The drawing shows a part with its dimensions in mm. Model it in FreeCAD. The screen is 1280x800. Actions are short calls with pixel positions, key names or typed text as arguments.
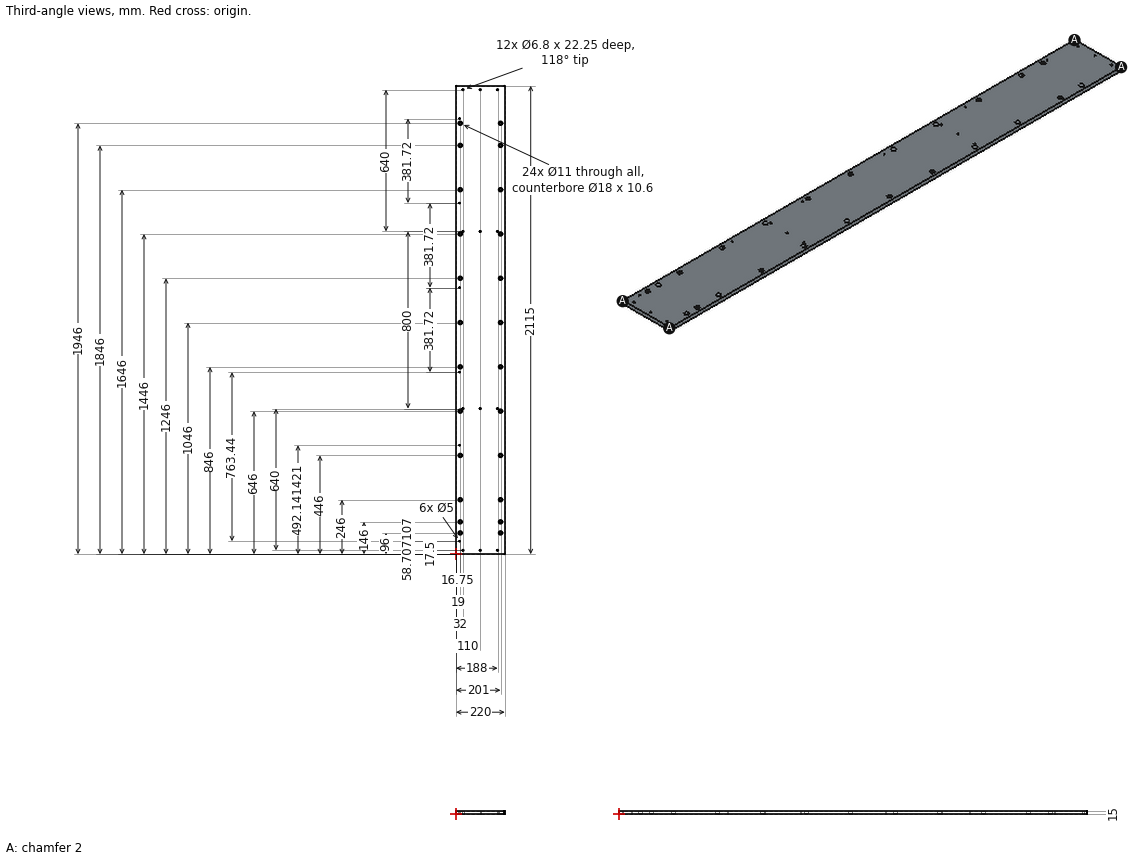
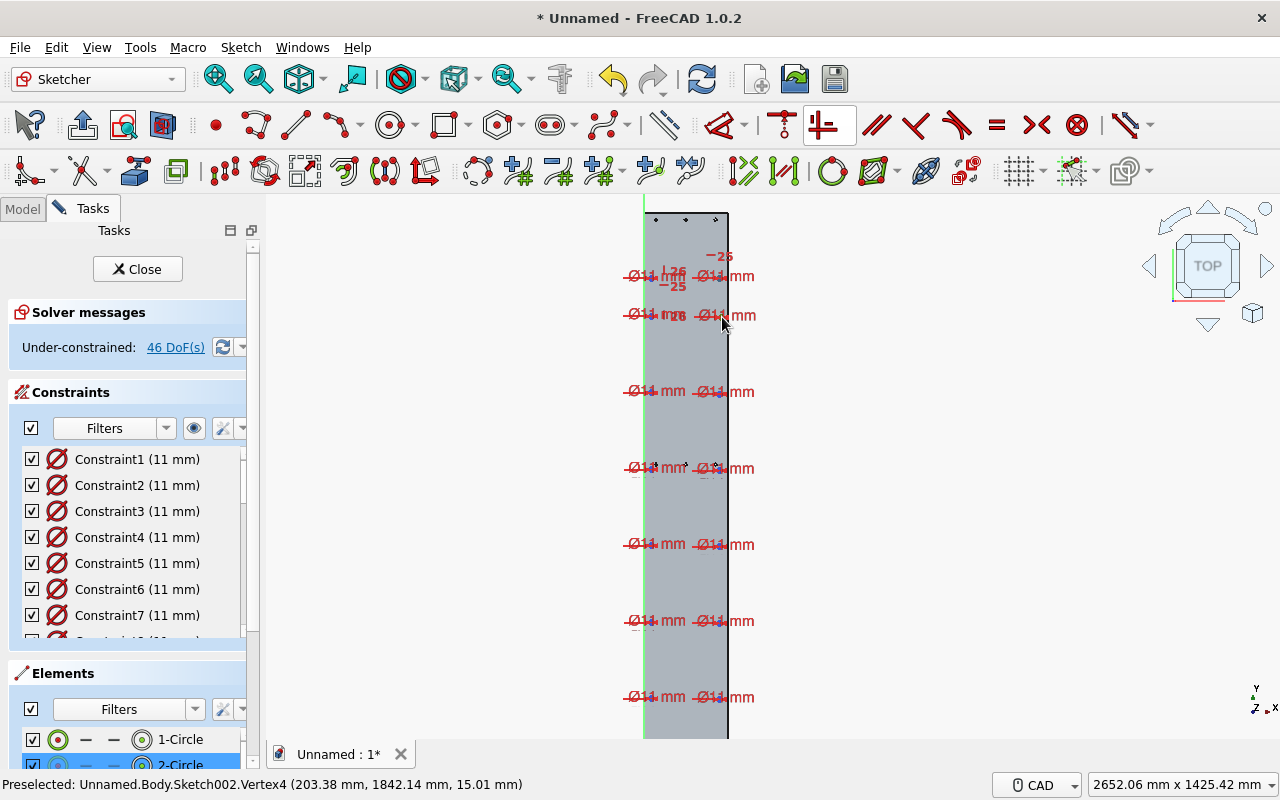
click(850, 126)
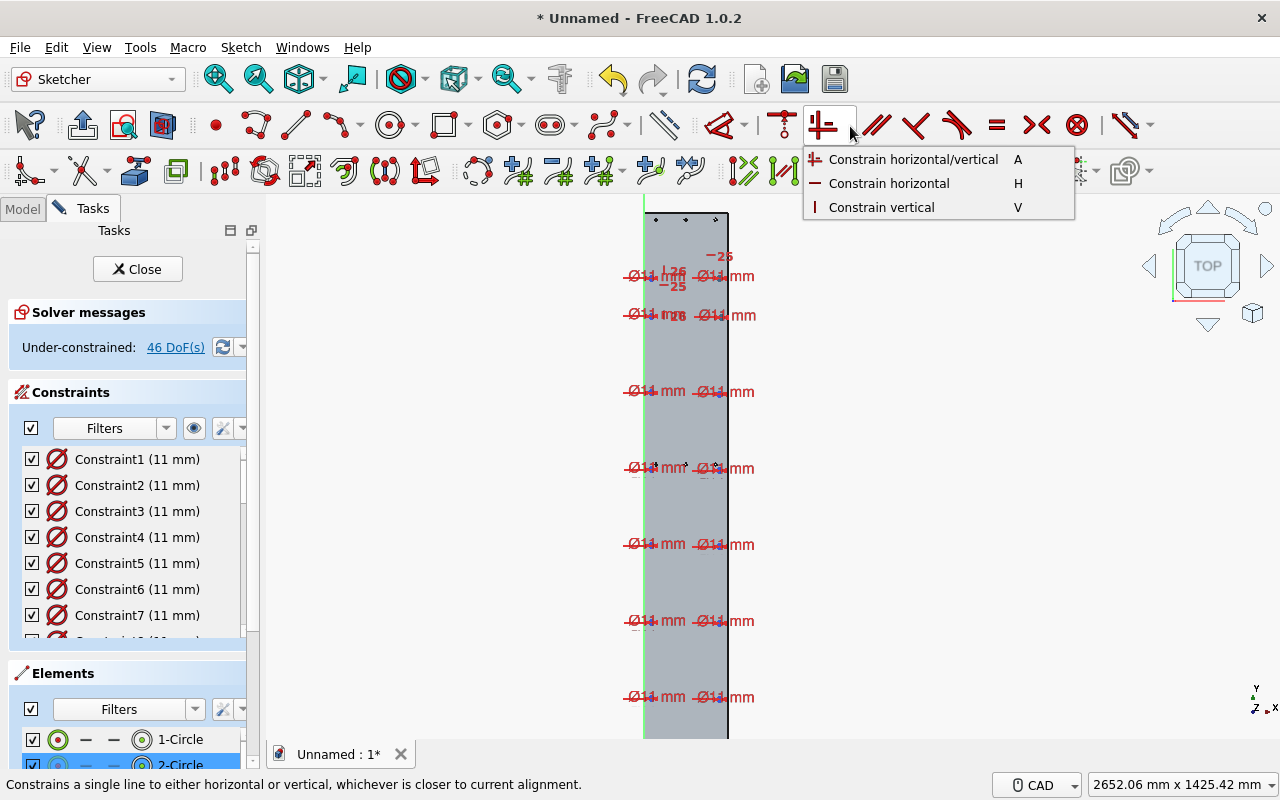
click(939, 207)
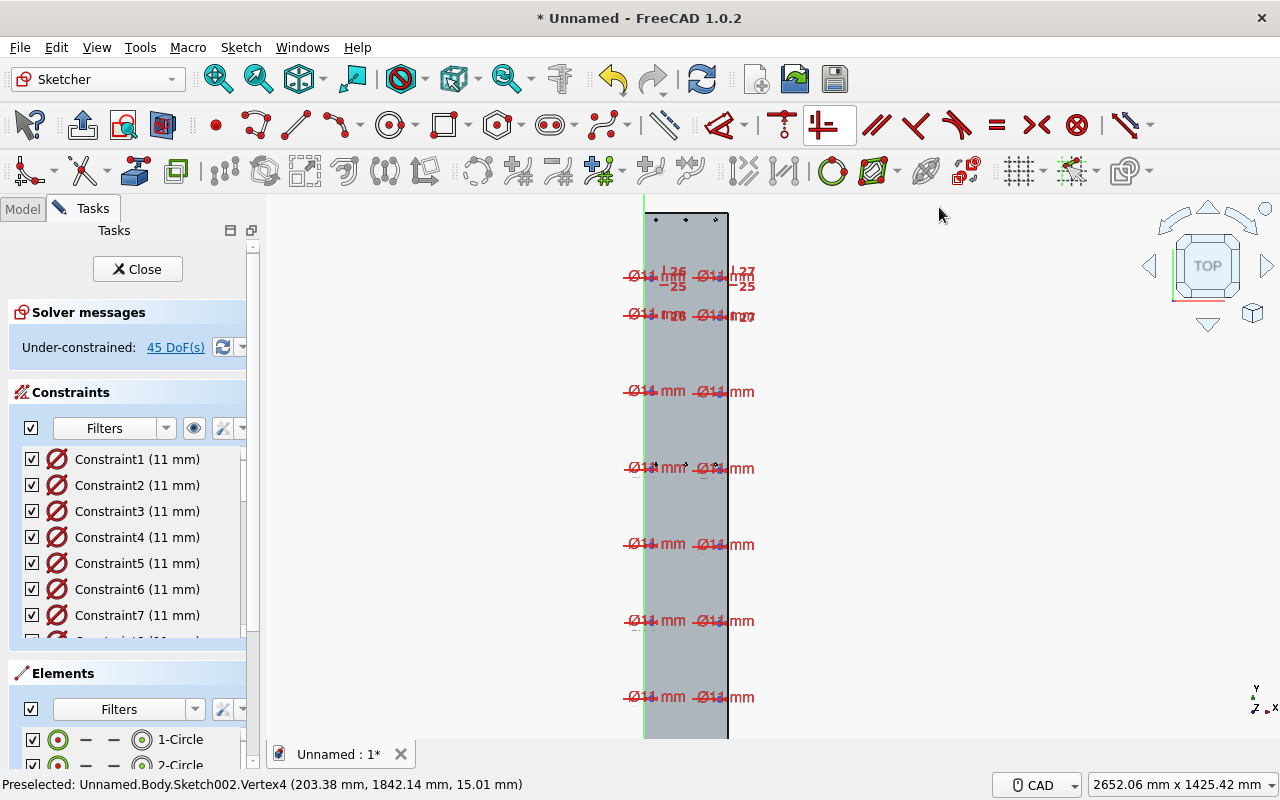
click(651, 316)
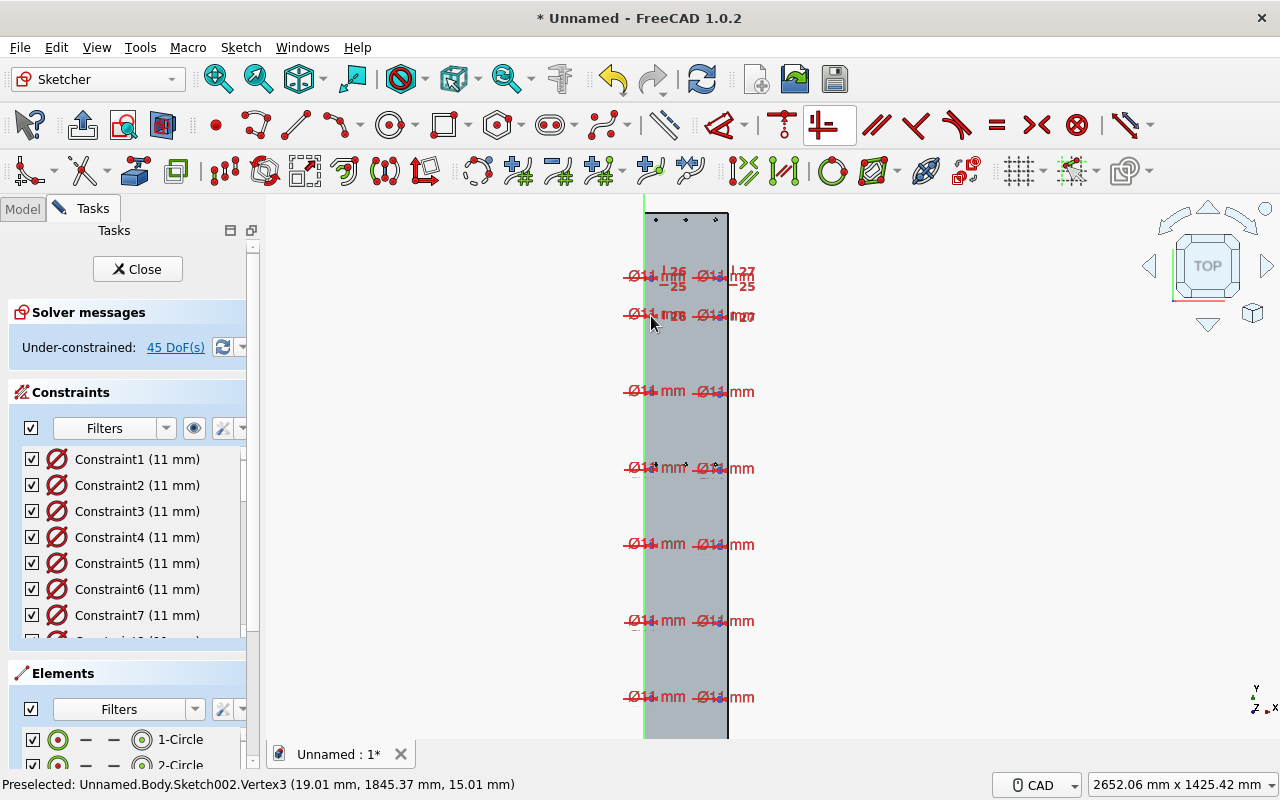
click(720, 317)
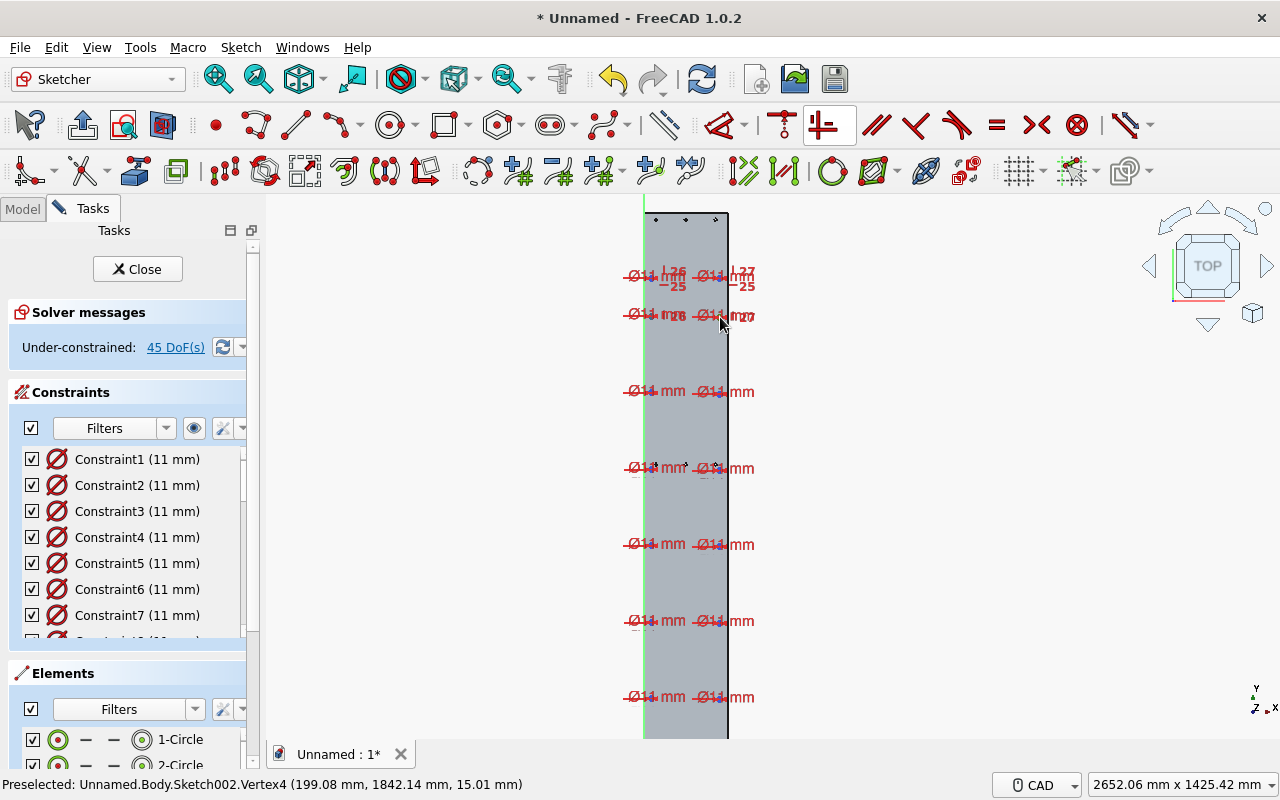
key(h)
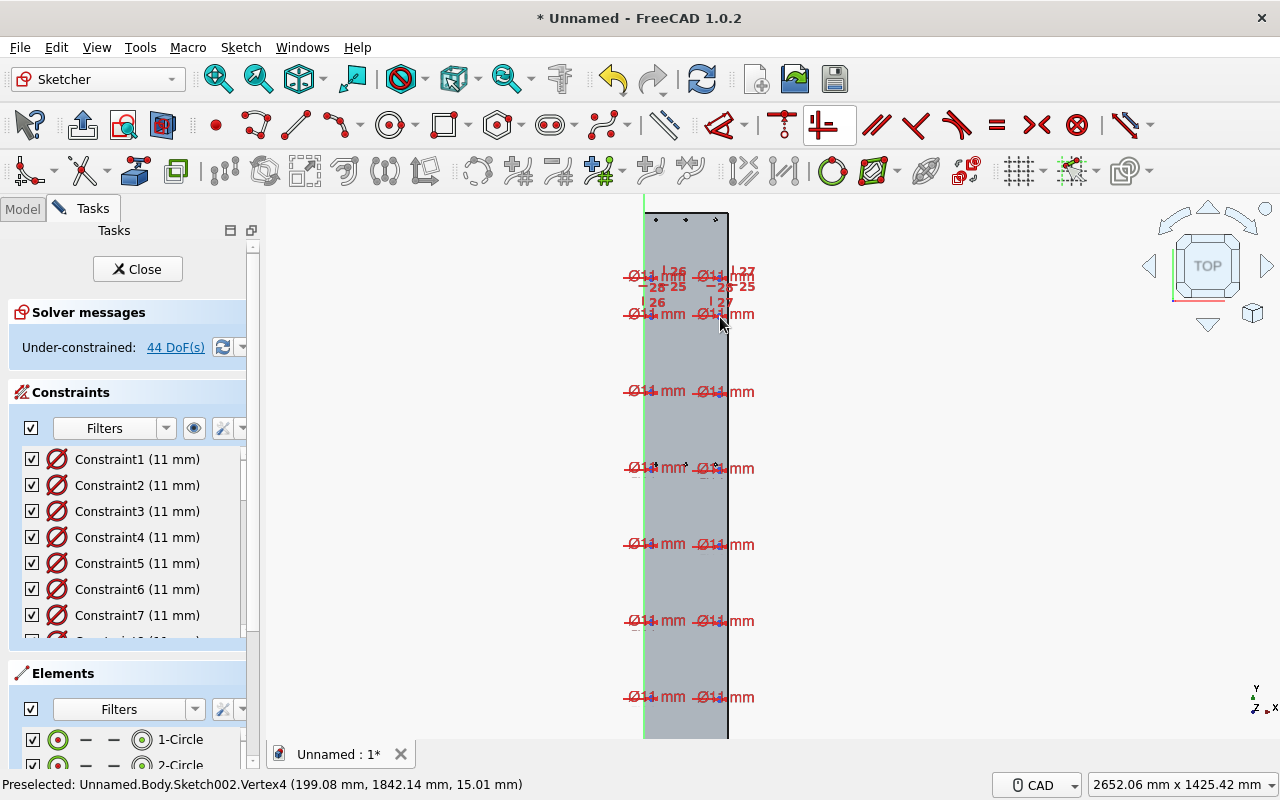
click(651, 316)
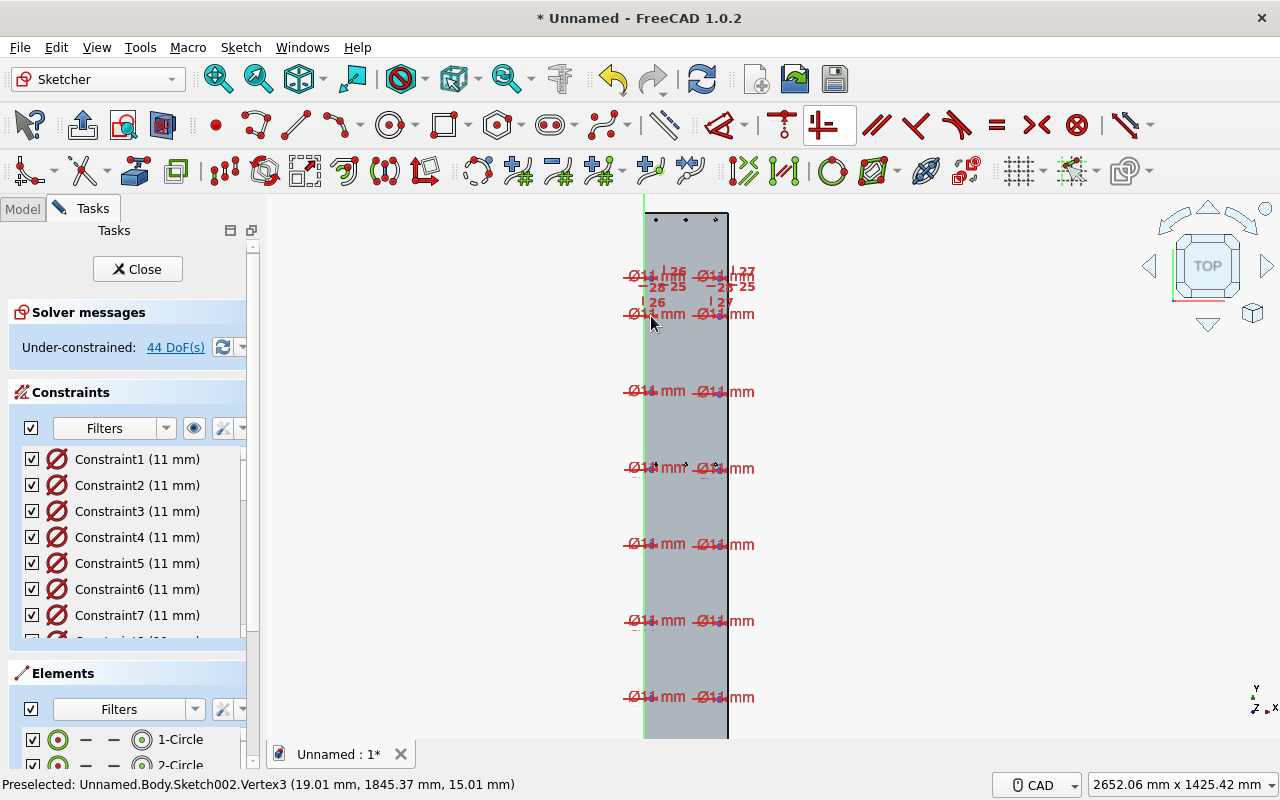
click(651, 393)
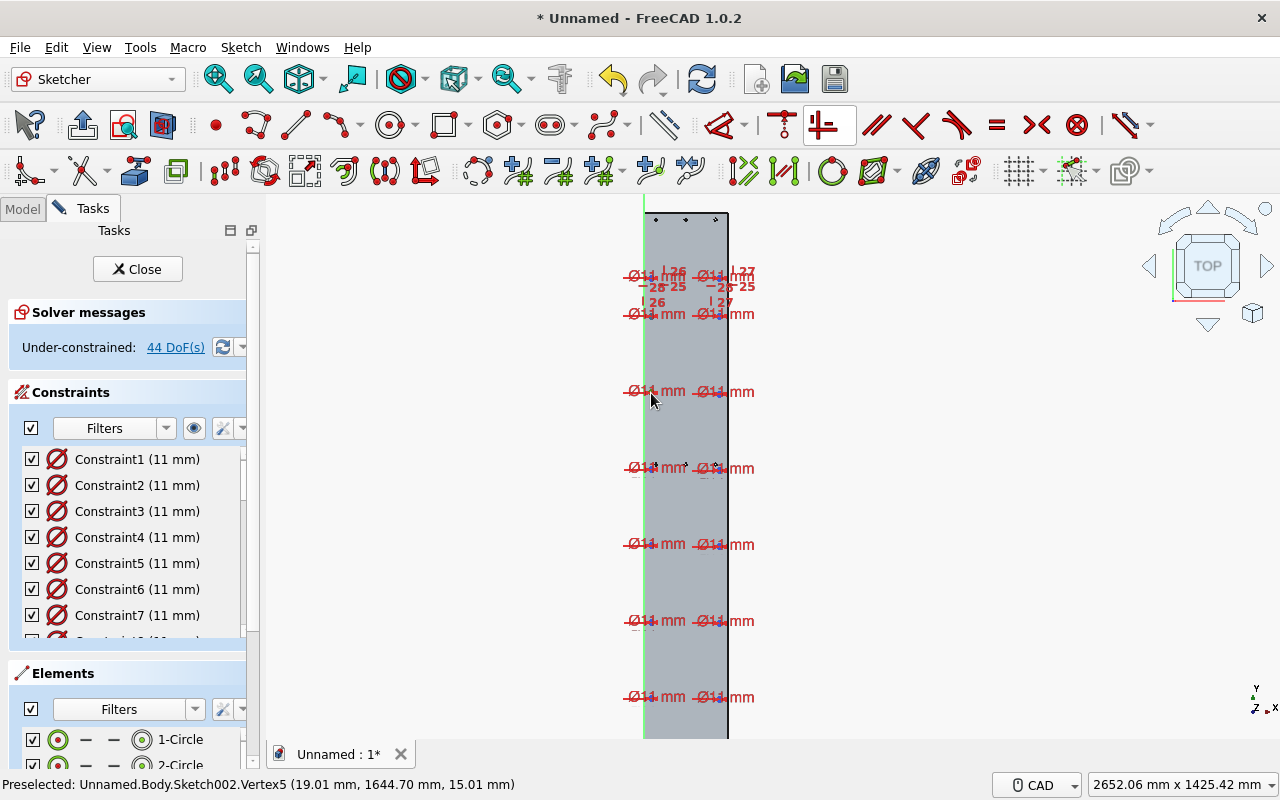
click(850, 126)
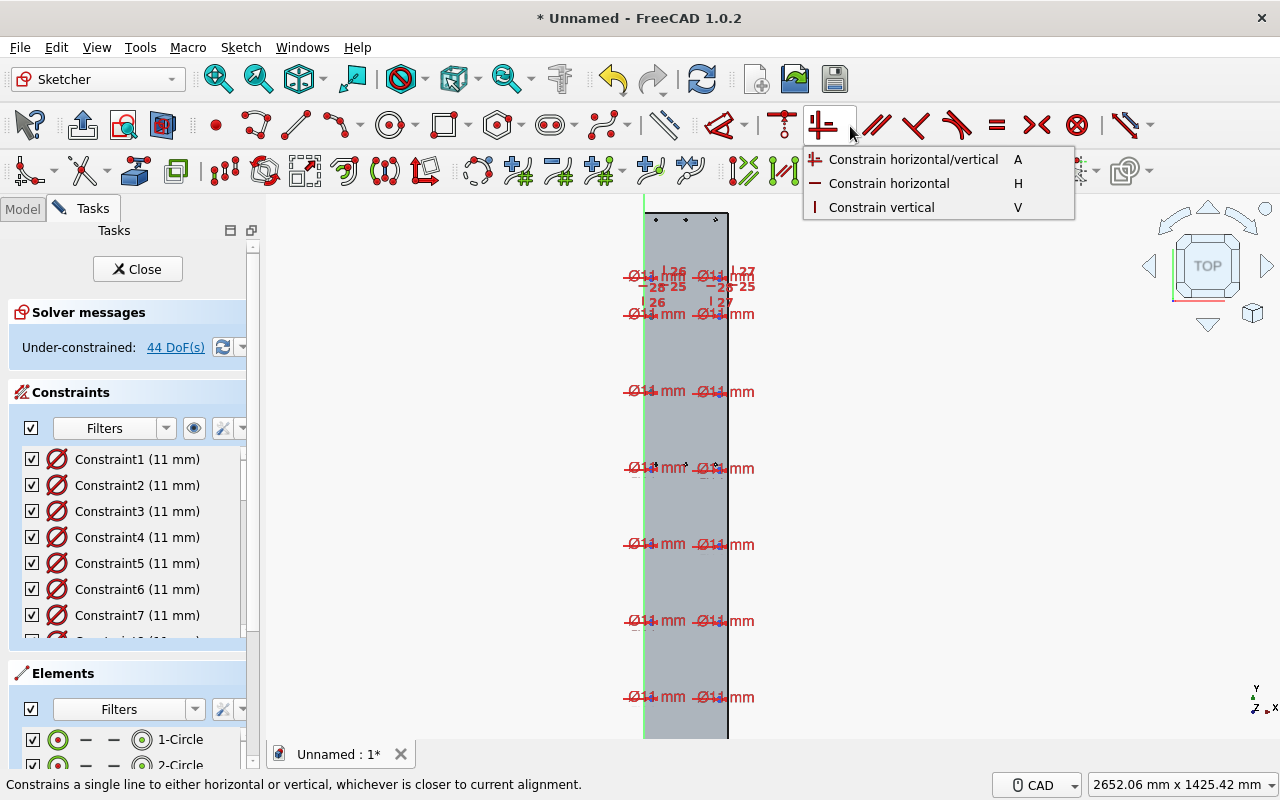
click(939, 207)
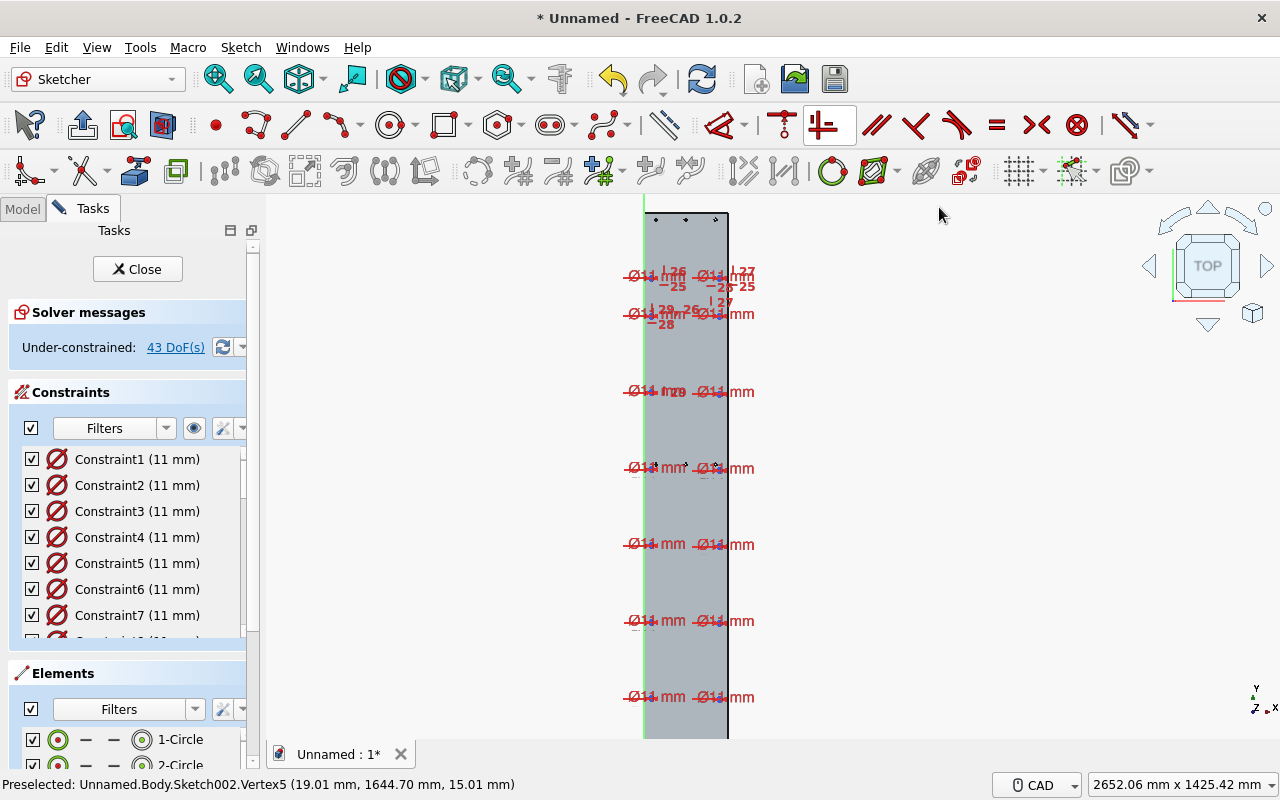
click(720, 316)